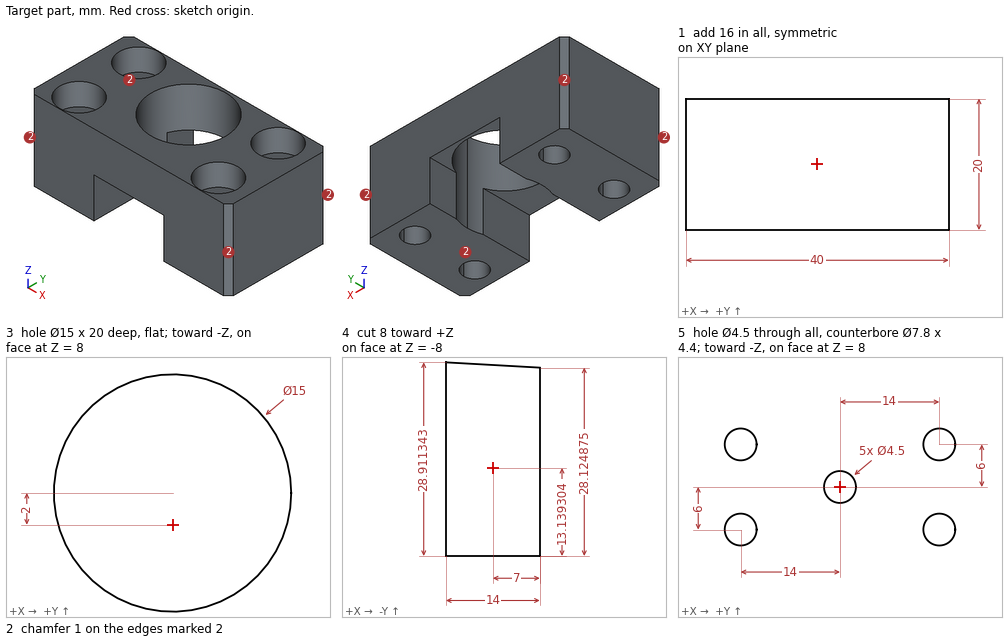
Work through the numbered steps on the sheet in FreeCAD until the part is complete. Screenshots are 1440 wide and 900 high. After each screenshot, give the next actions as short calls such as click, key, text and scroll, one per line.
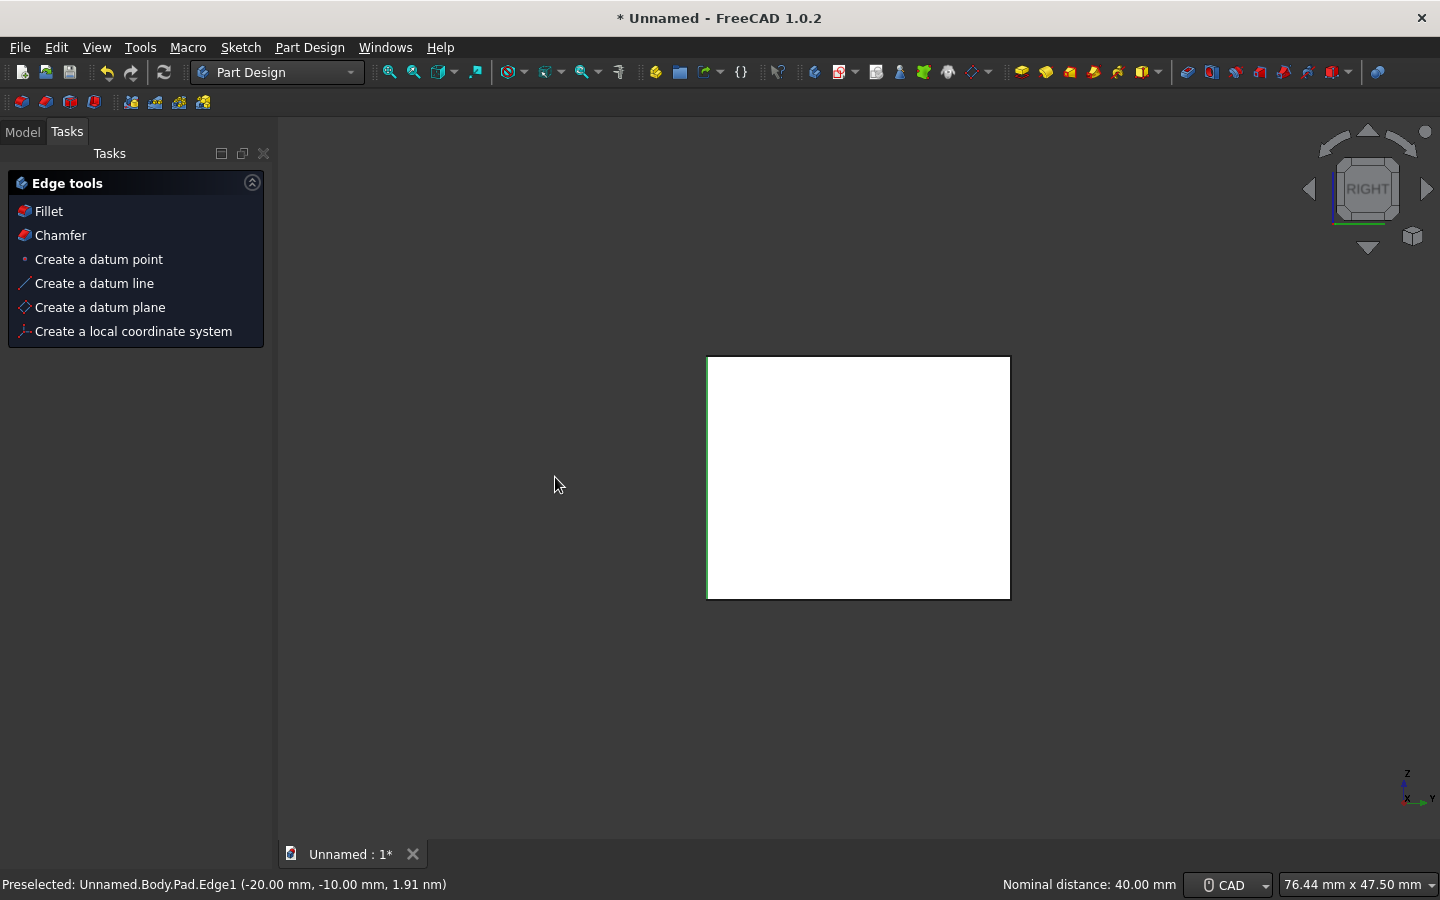
key(v)
key(f)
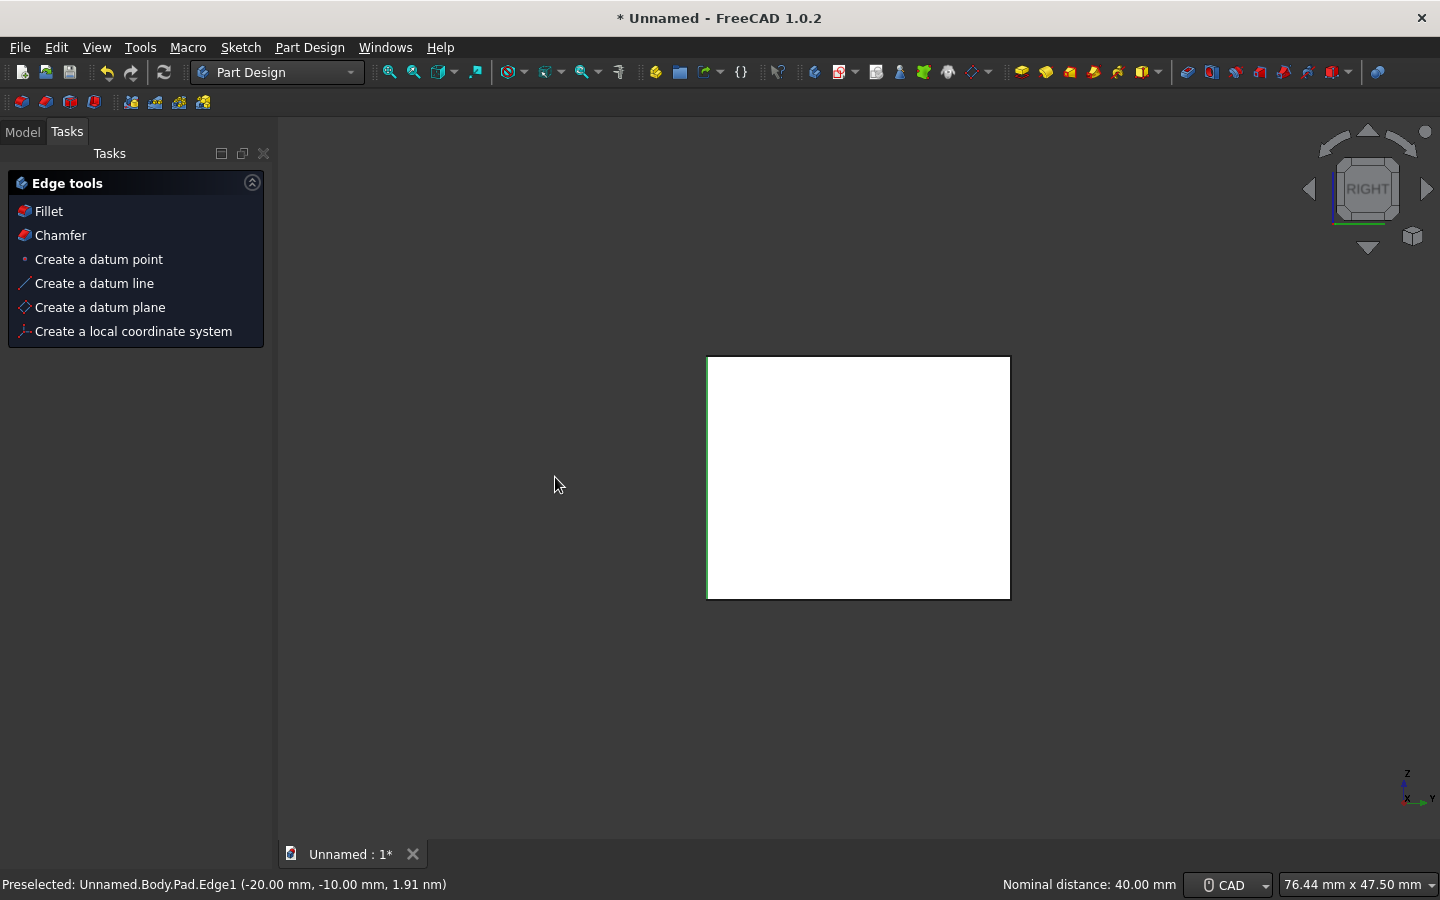
click(1011, 477, ctrl)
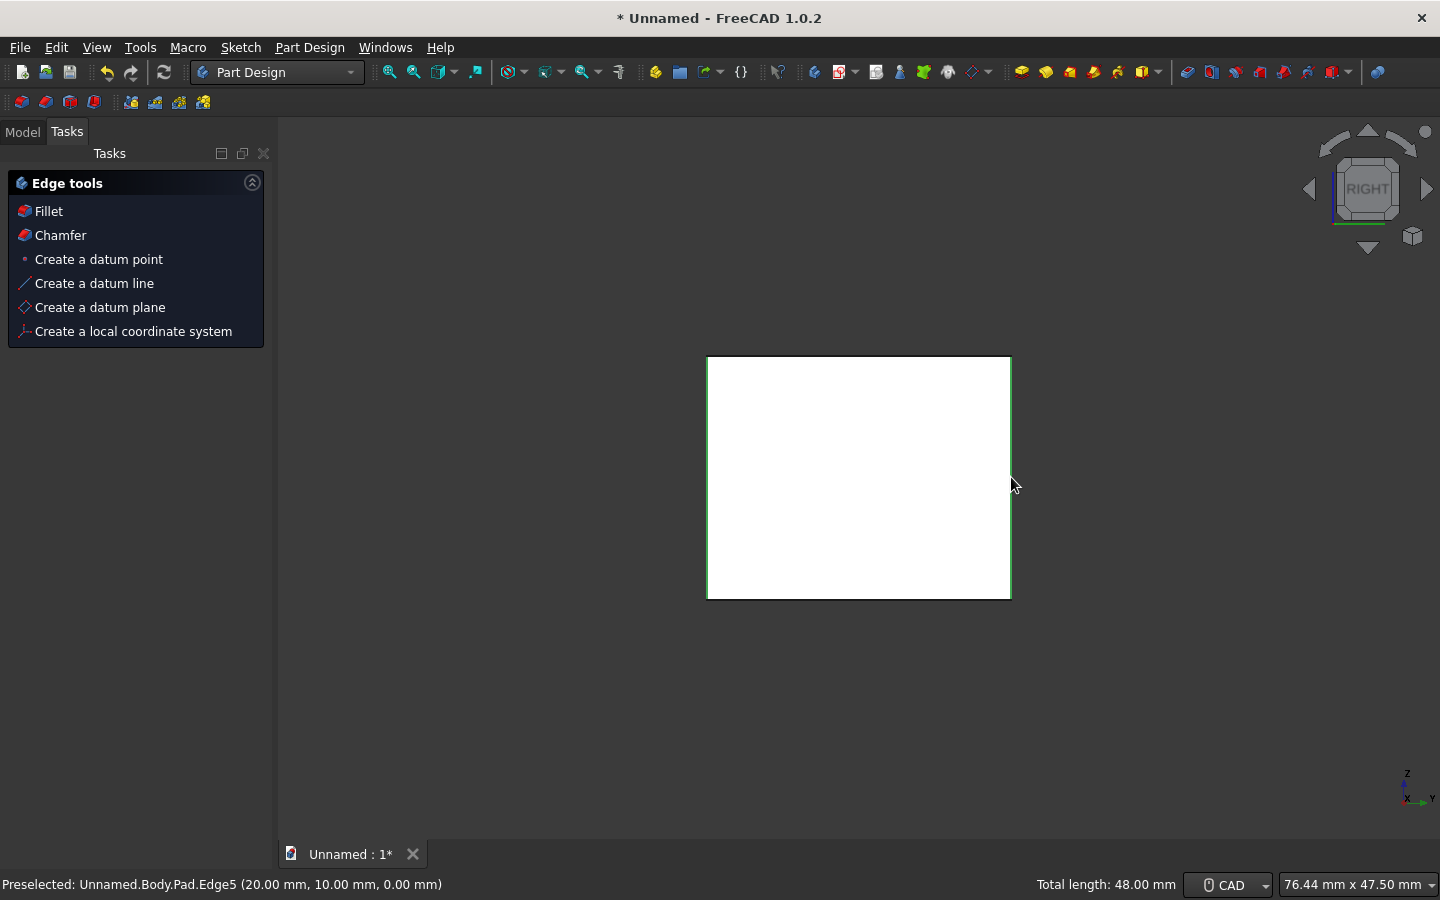
key(5)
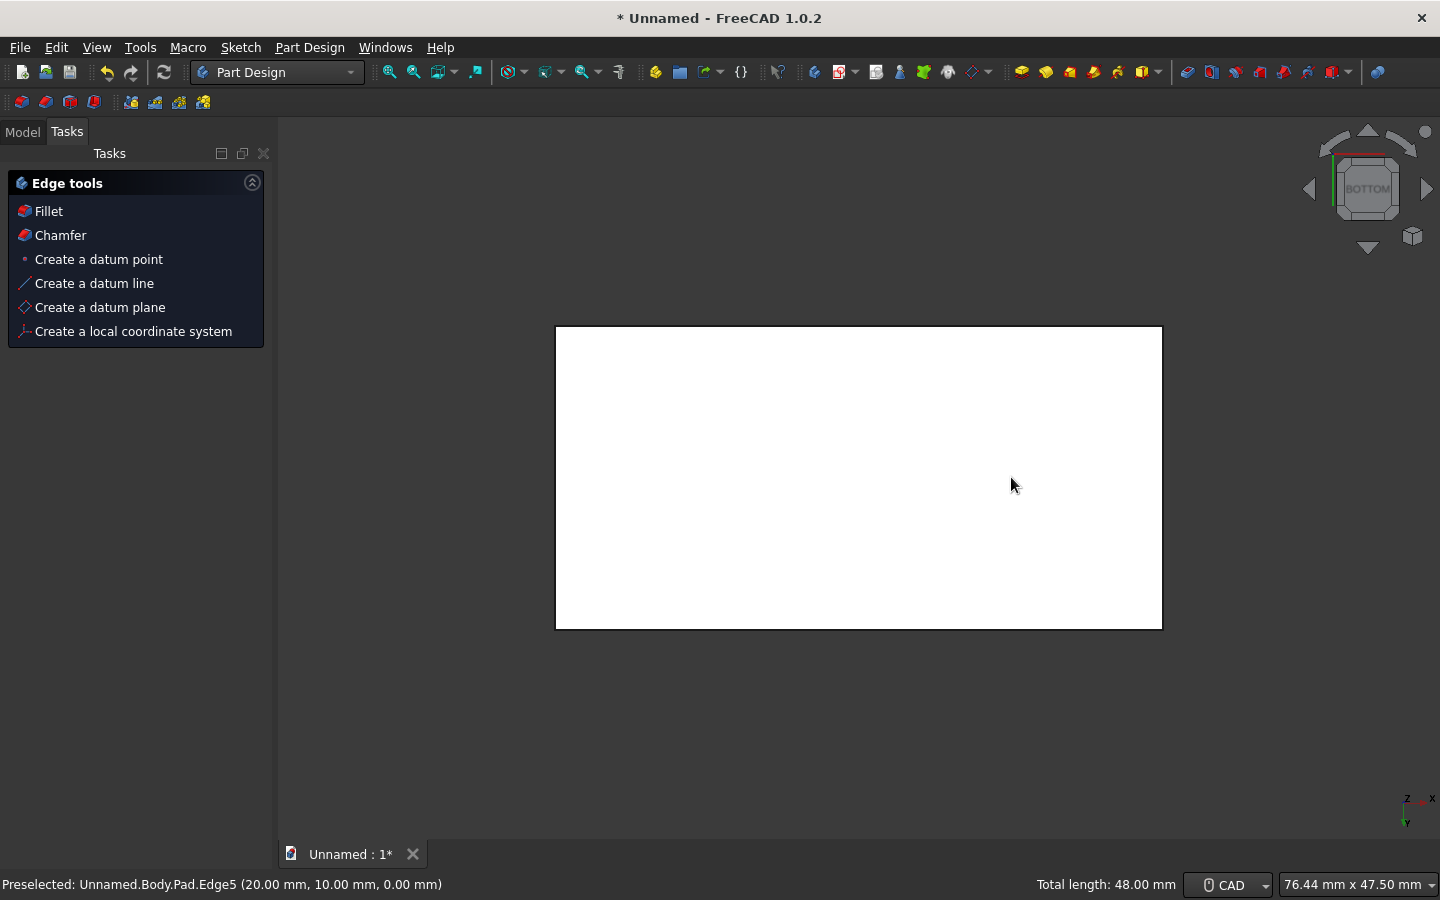
key(4)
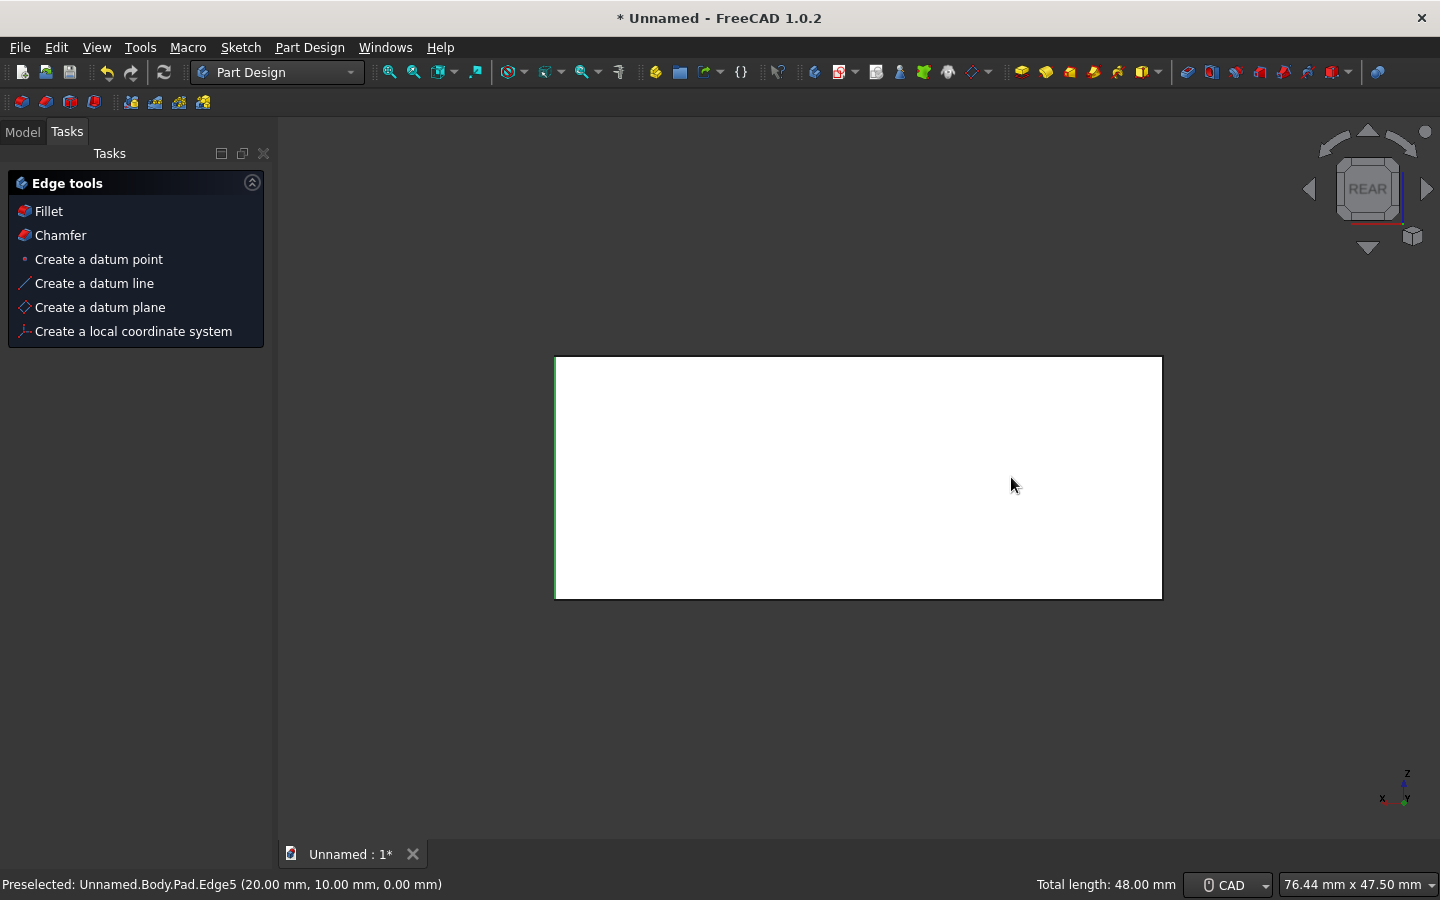
click(1163, 477, ctrl)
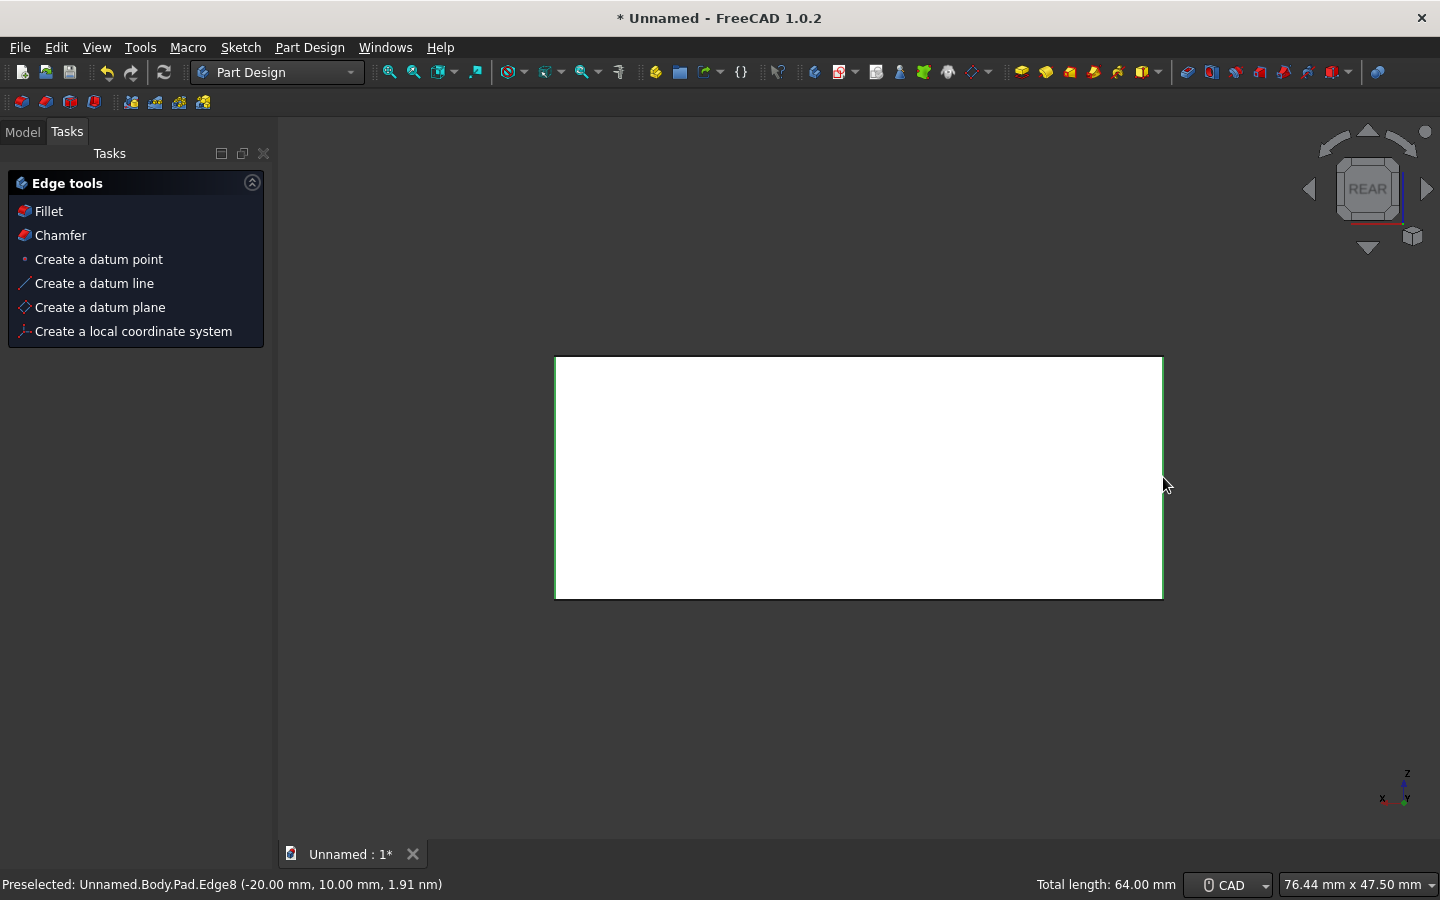
click(46, 102)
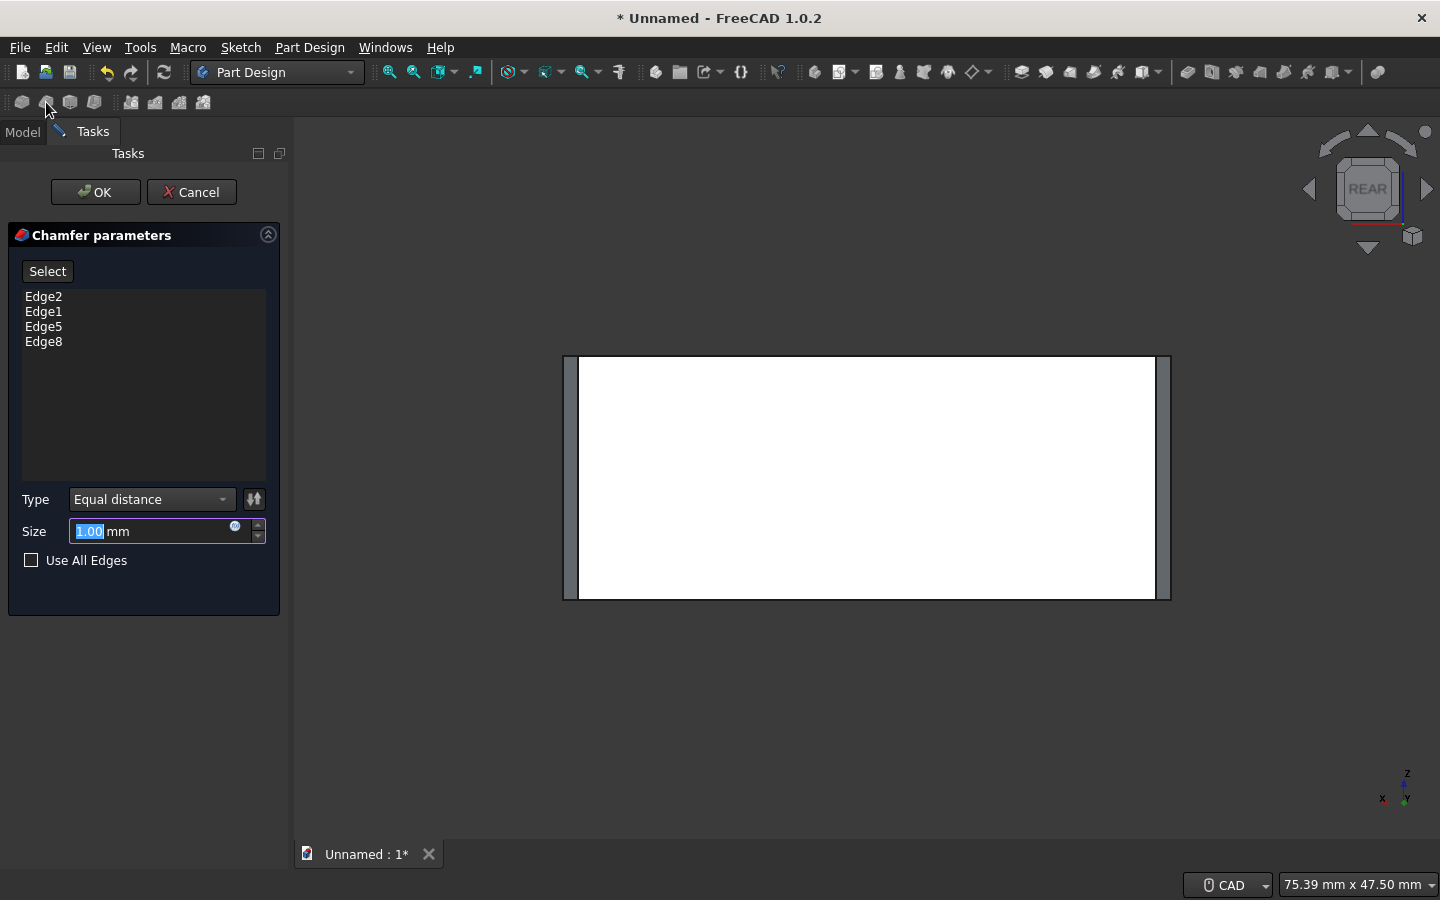
text(1)
key(Tab)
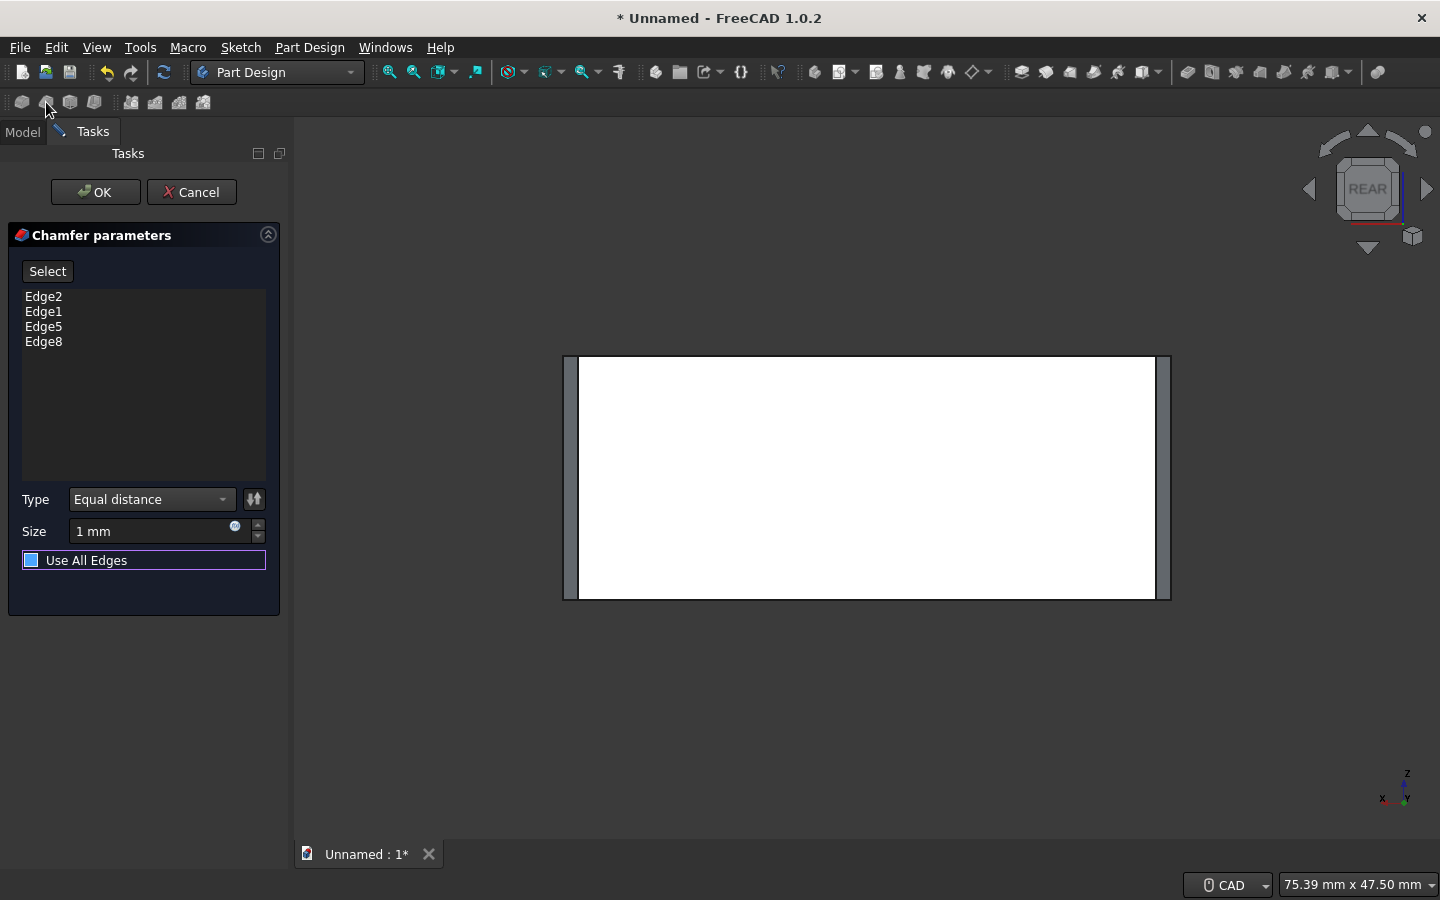
click(96, 192)